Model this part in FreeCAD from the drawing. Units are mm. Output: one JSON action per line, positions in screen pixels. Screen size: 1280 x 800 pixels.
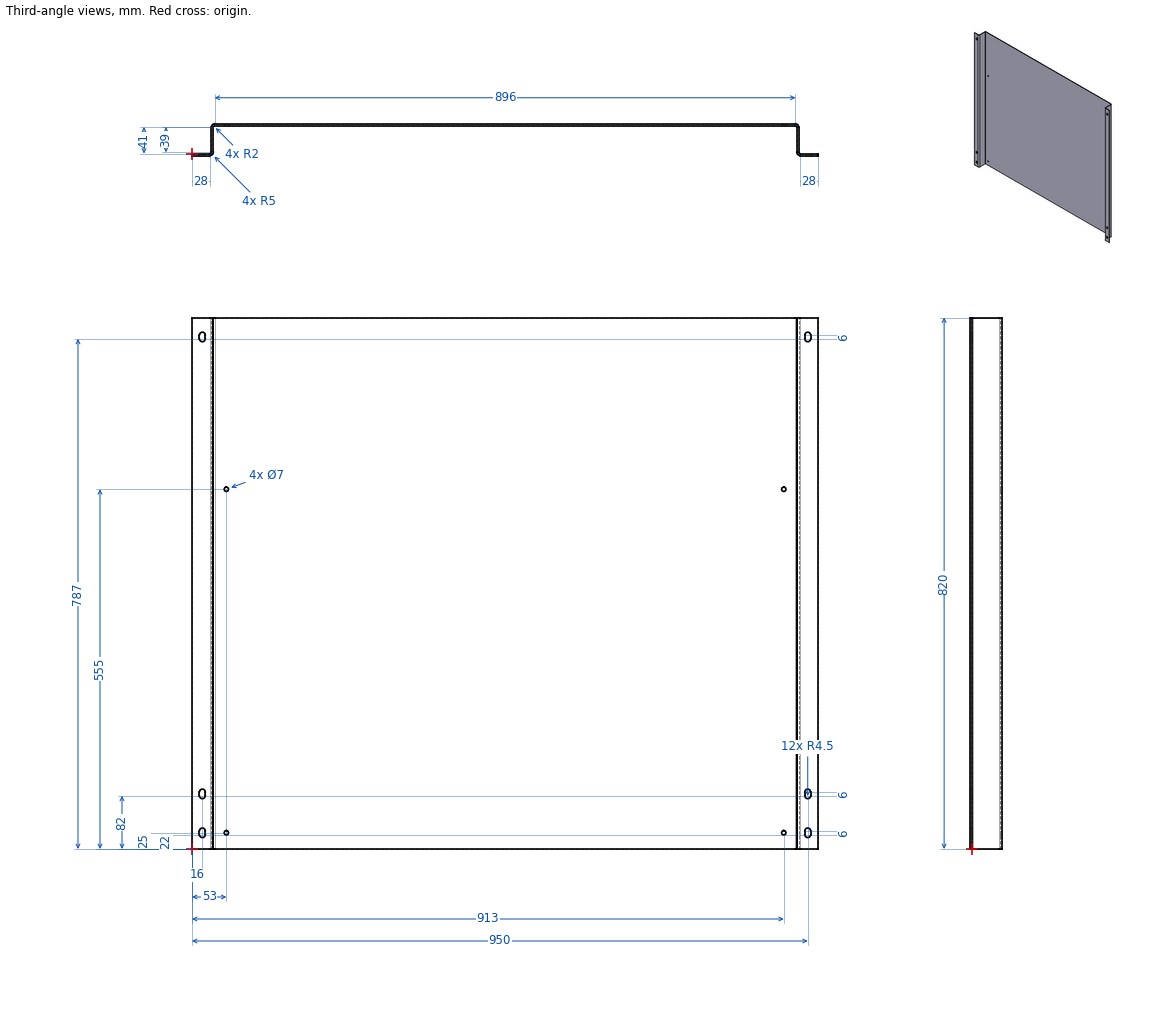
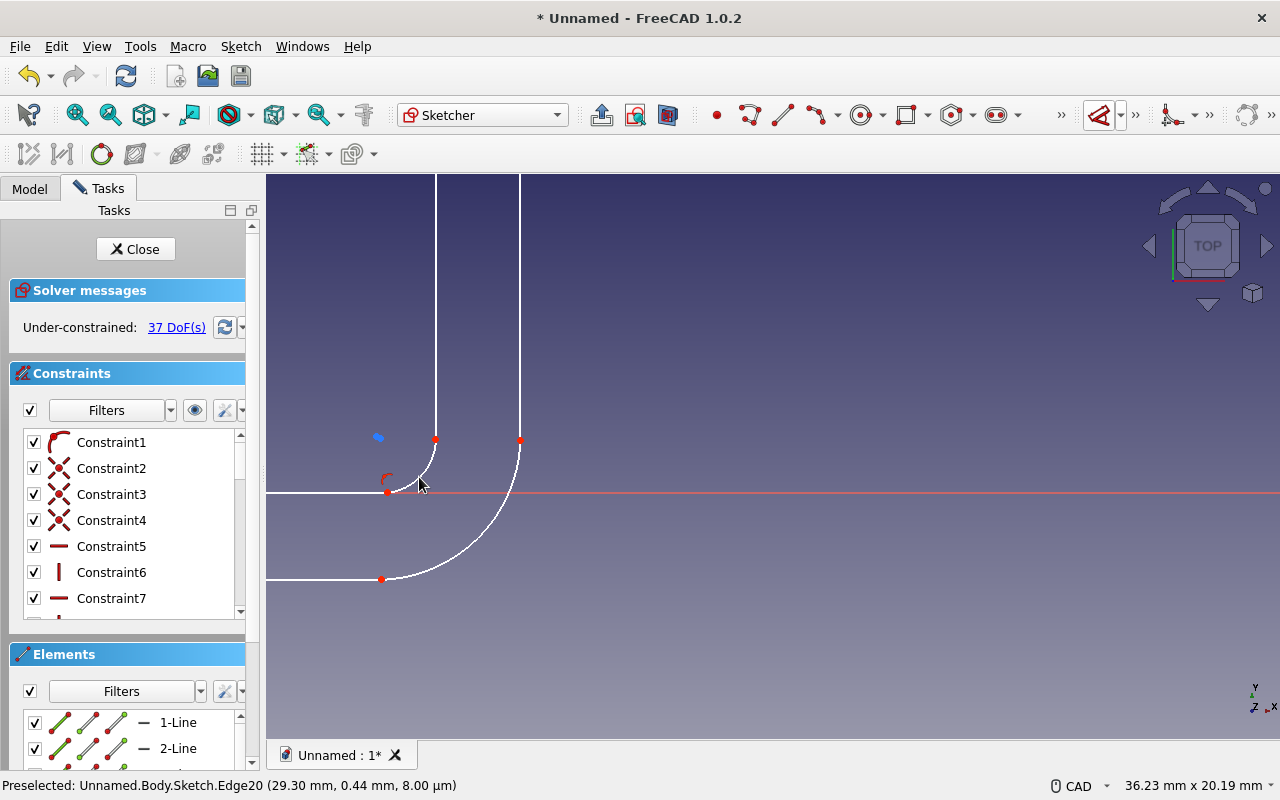
{"action": "scroll", "coordinate": [356, 472], "scroll_direction": "down", "scroll_amount": 18}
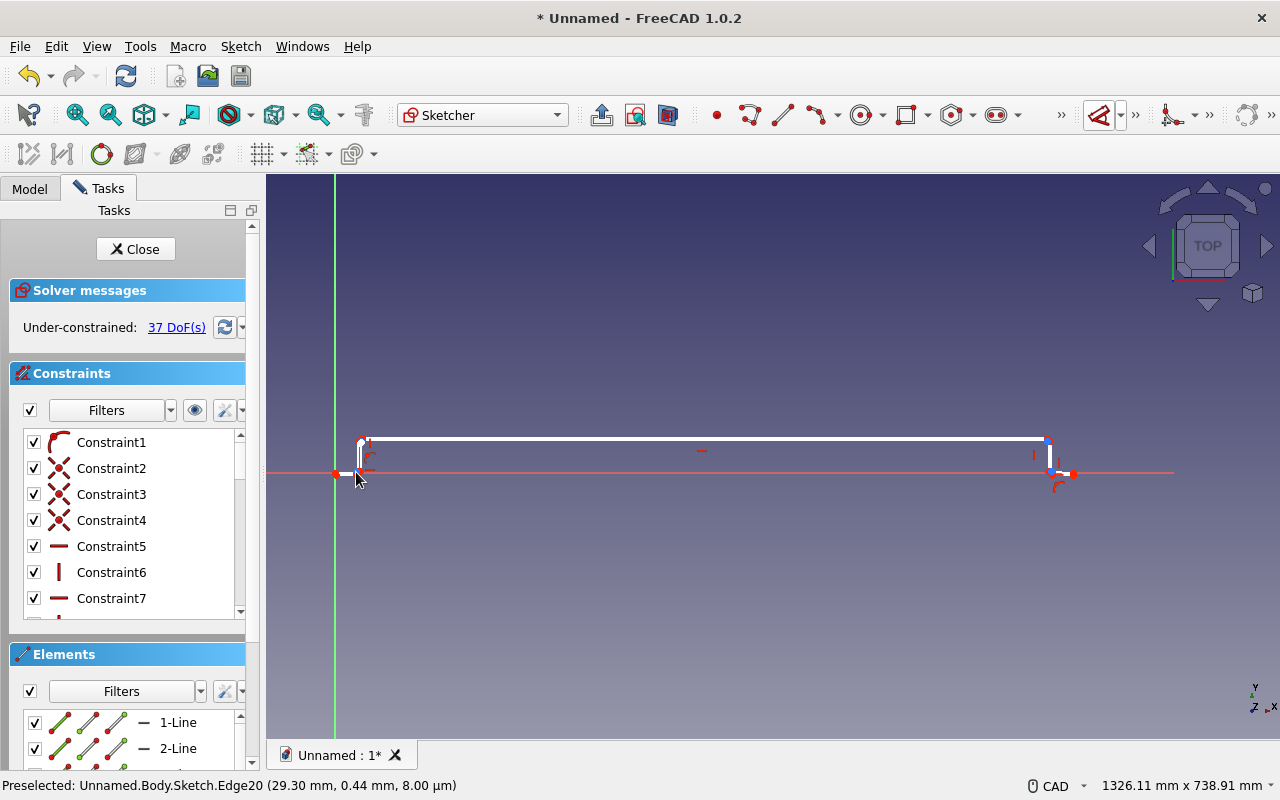
{"action": "scroll", "coordinate": [350, 473], "scroll_direction": "up", "scroll_amount": 9}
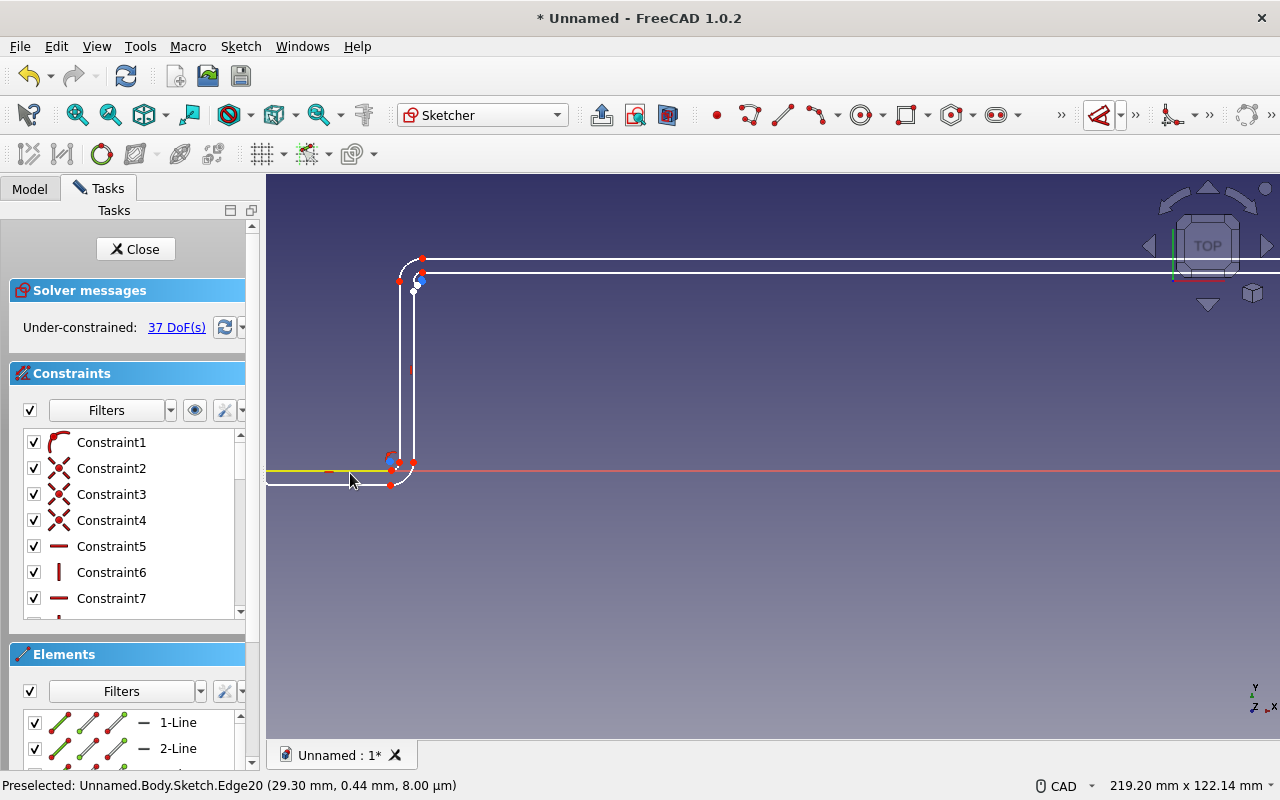
{"action": "left_click", "coordinate": [352, 471]}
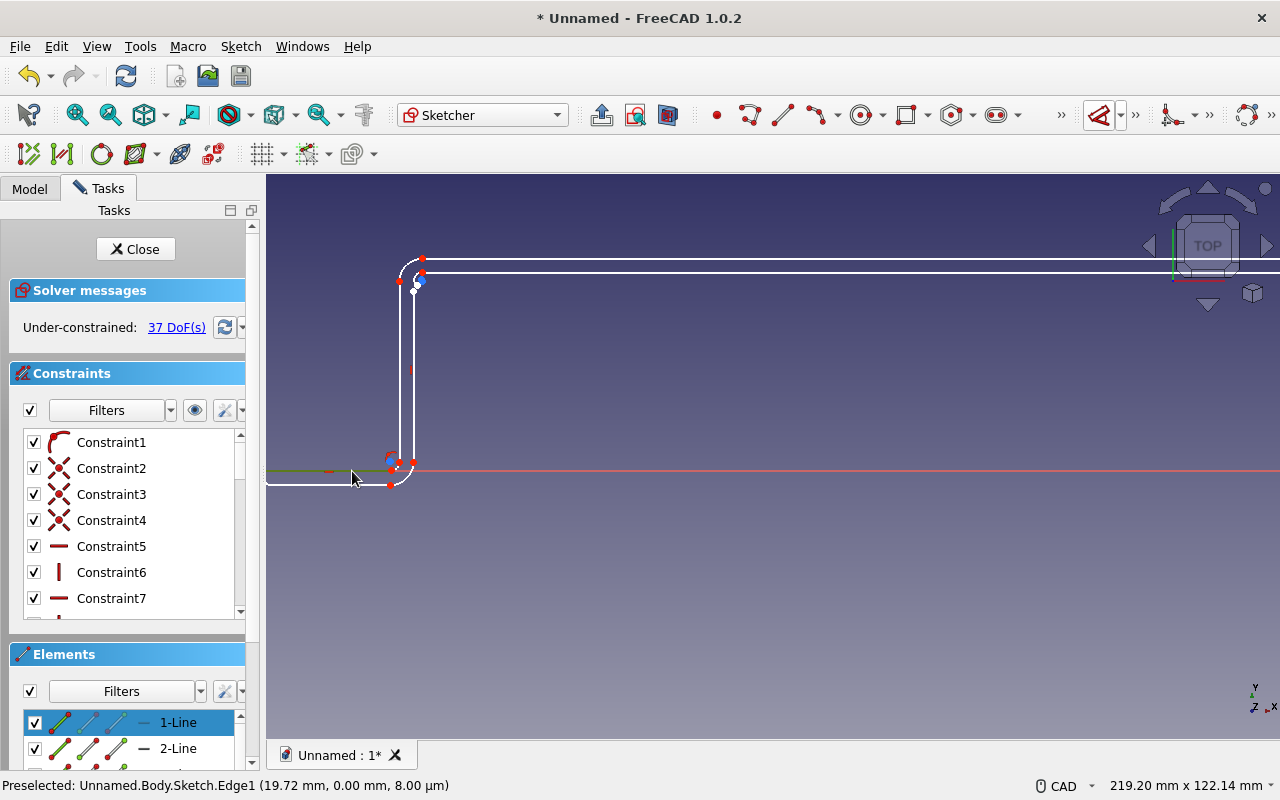
{"action": "scroll", "coordinate": [397, 468], "scroll_direction": "up", "scroll_amount": 4}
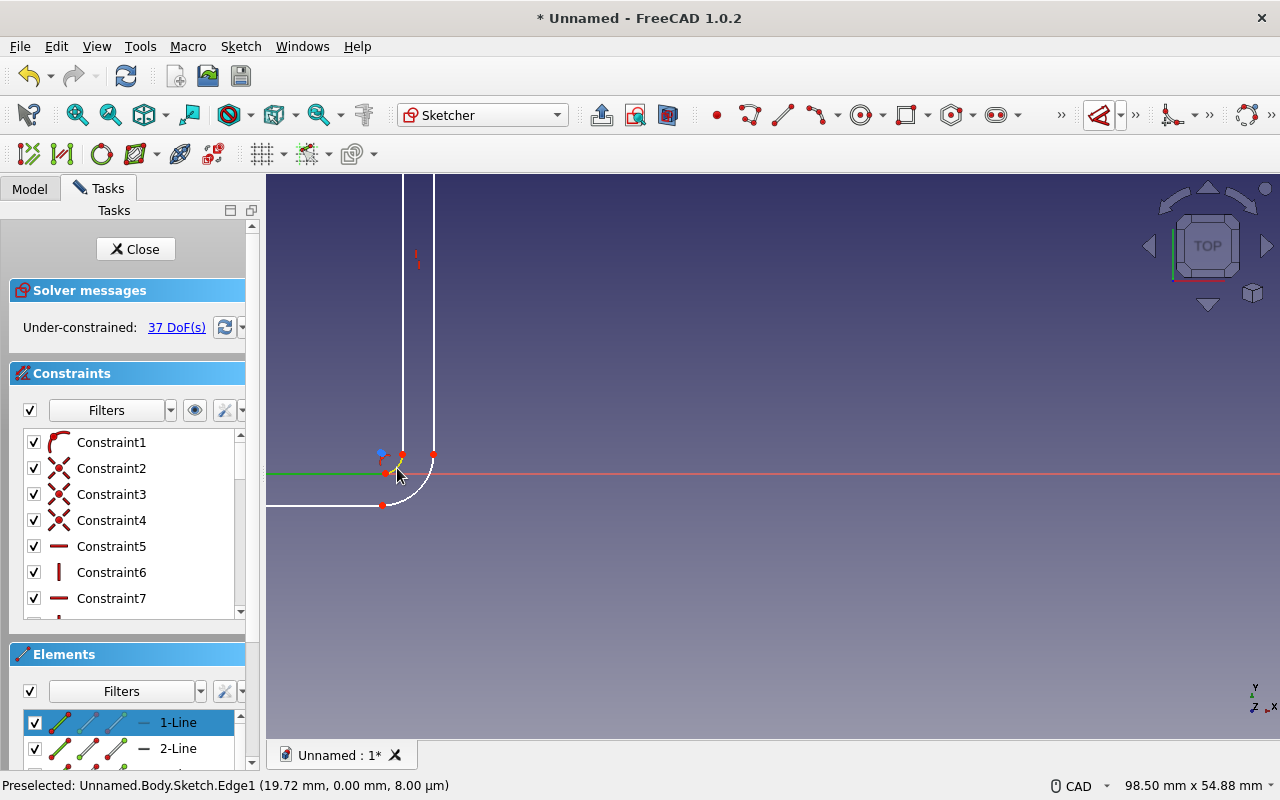
{"action": "left_click", "coordinate": [397, 467]}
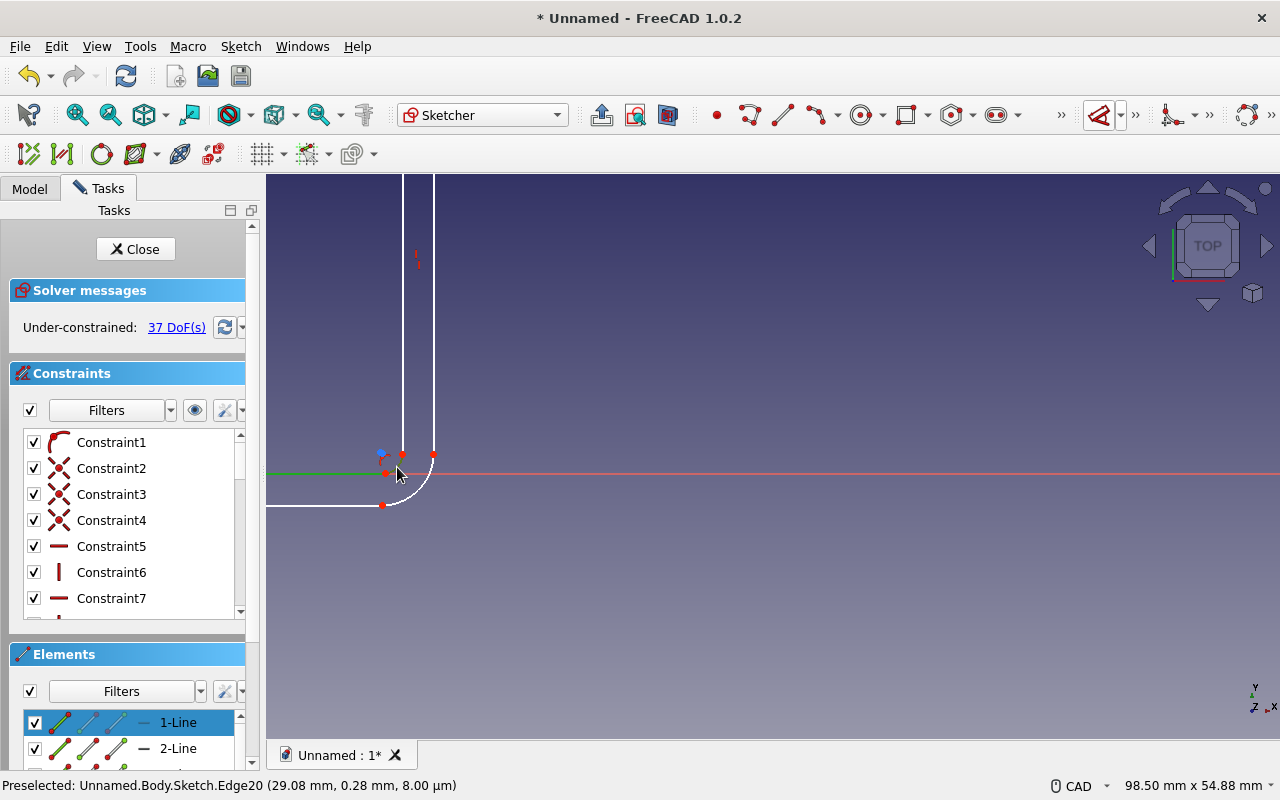
{"action": "key", "text": "t"}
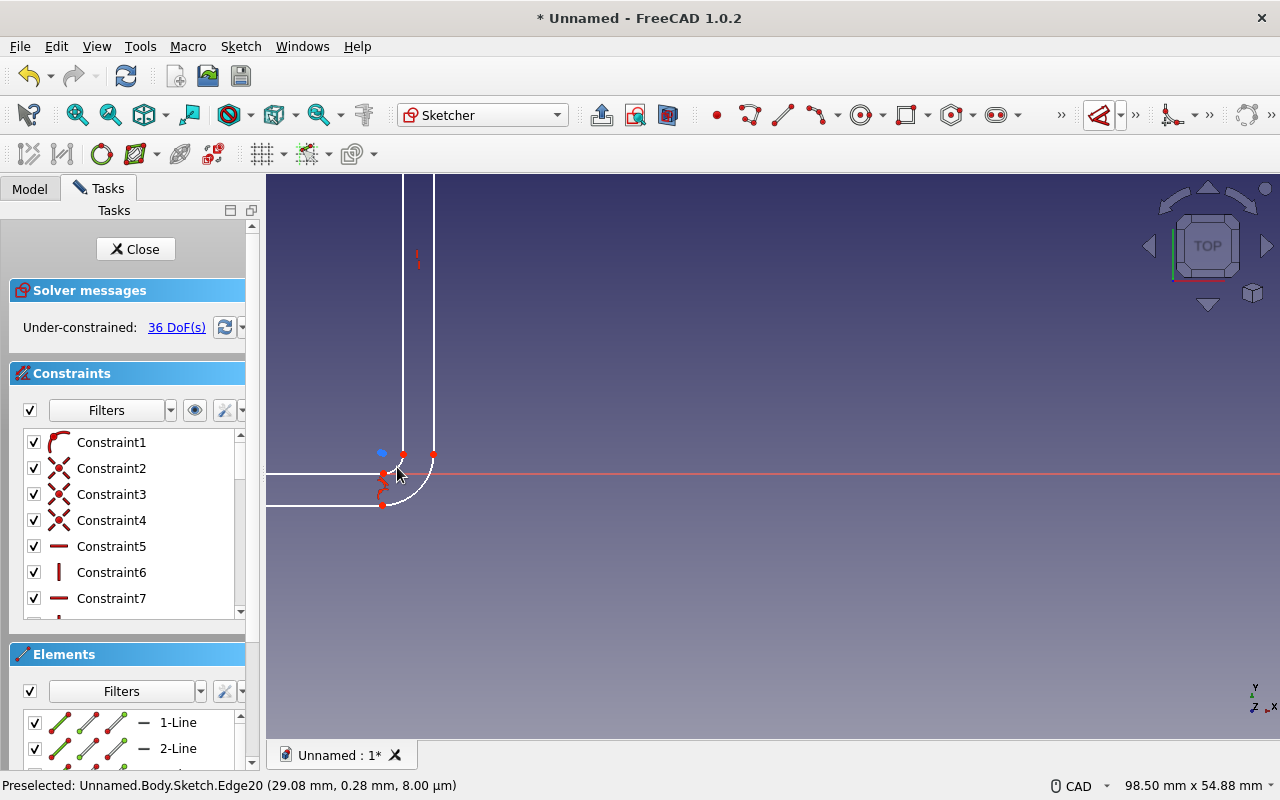
{"action": "left_click", "coordinate": [301, 506]}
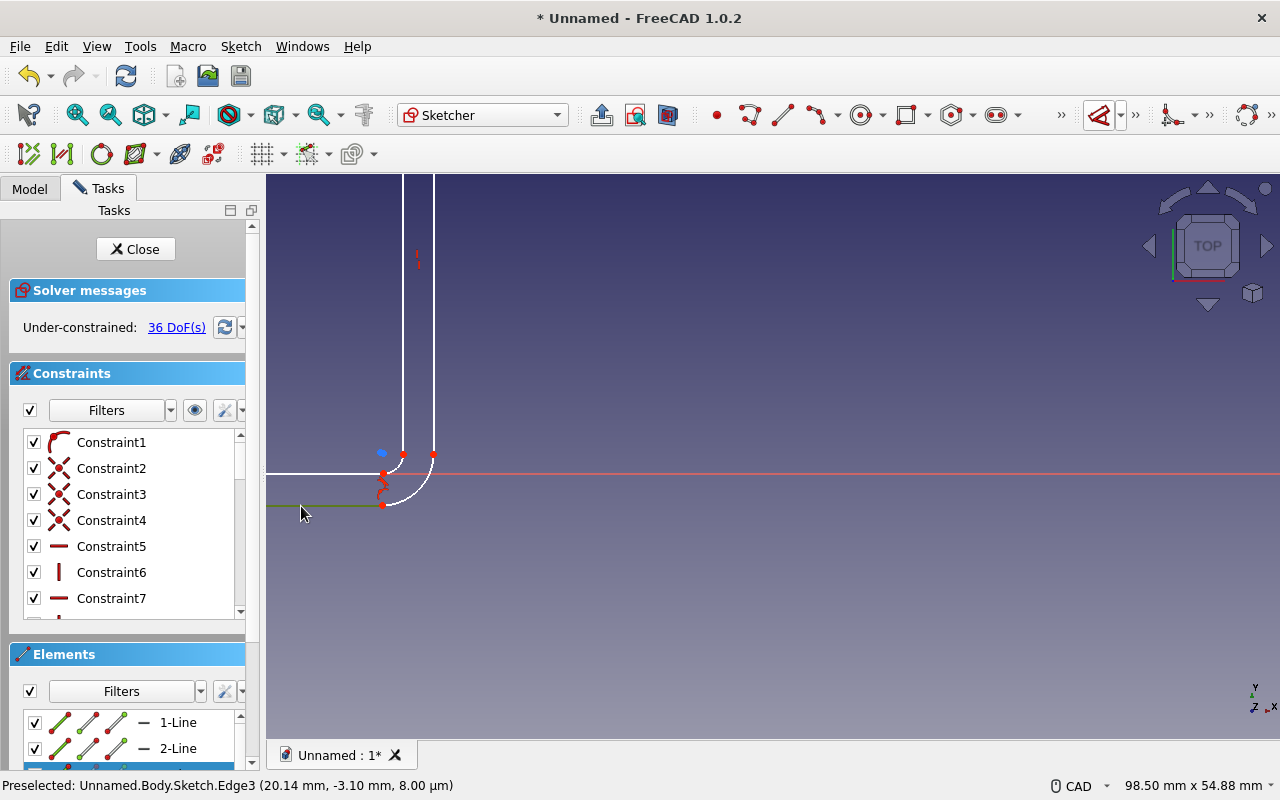
{"action": "left_click", "coordinate": [405, 500]}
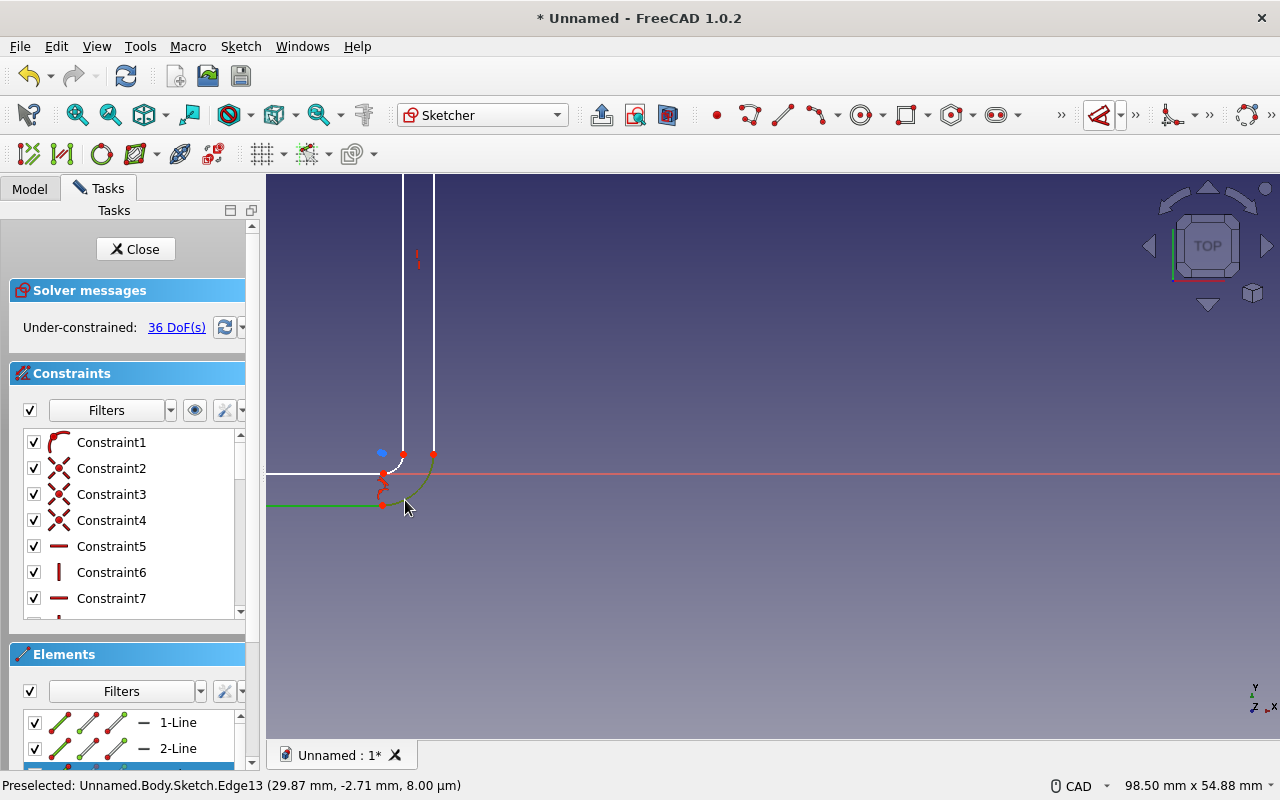
{"action": "key", "text": "t"}